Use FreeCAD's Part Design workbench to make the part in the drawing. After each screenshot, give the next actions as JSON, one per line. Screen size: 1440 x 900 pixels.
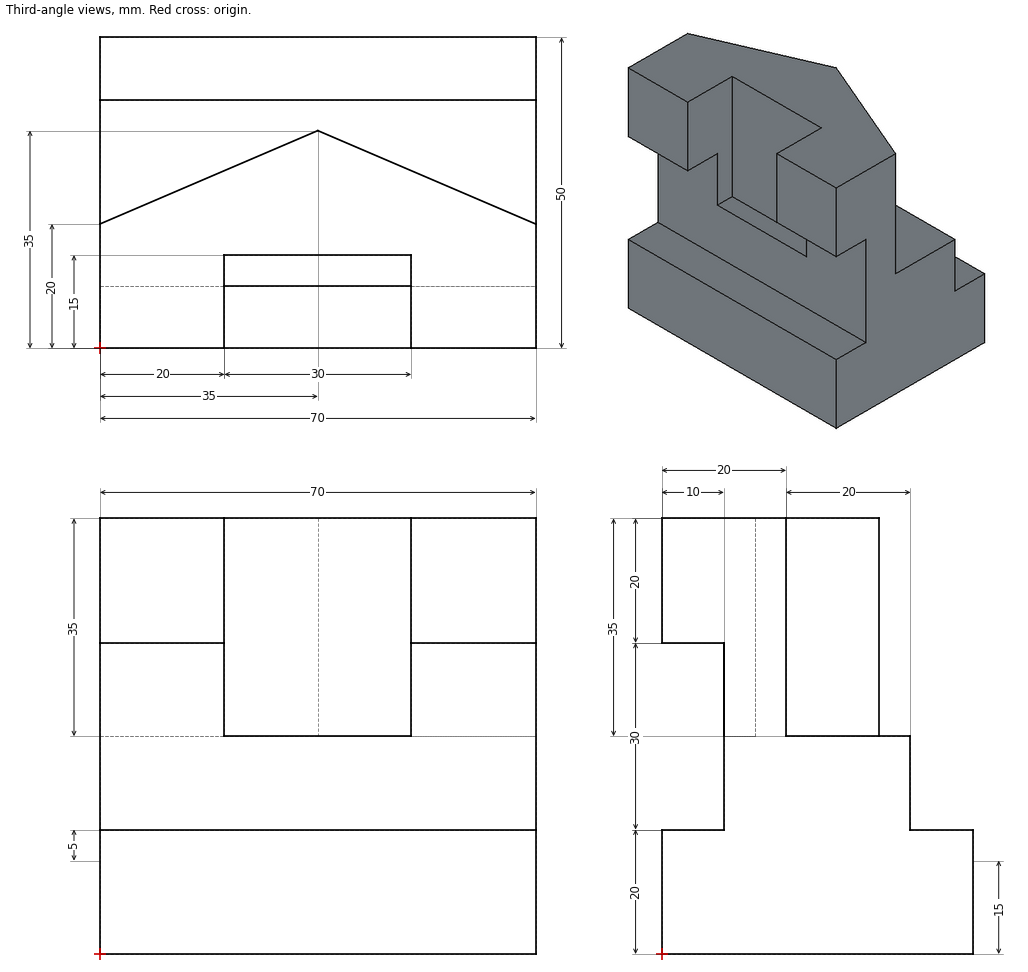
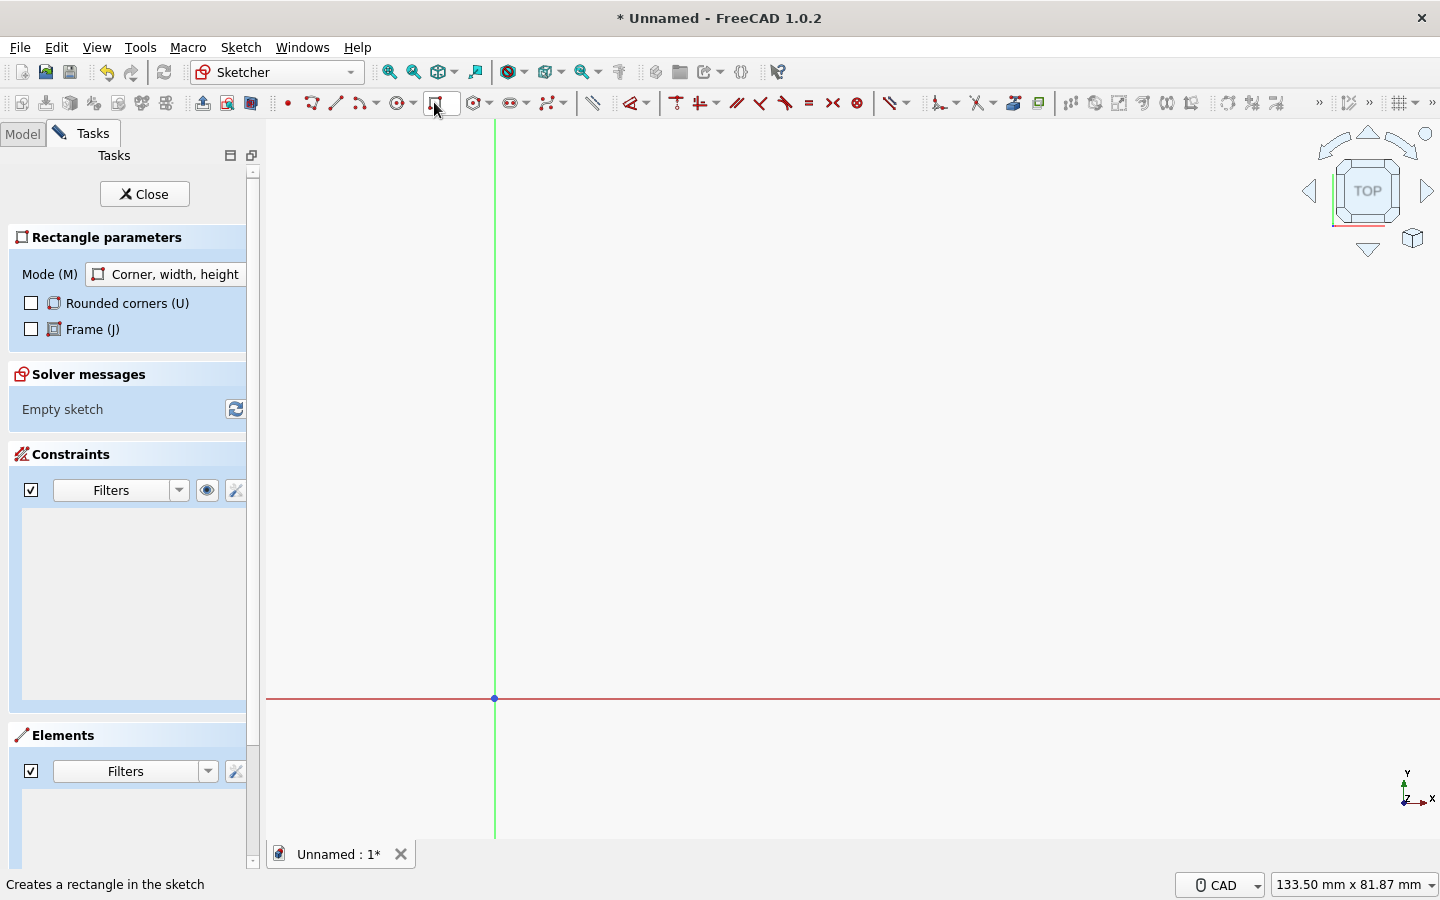
{"action": "left_click", "coordinate": [495, 699]}
{"action": "left_click", "coordinate": [1110, 259]}
{"action": "key", "text": "Escape"}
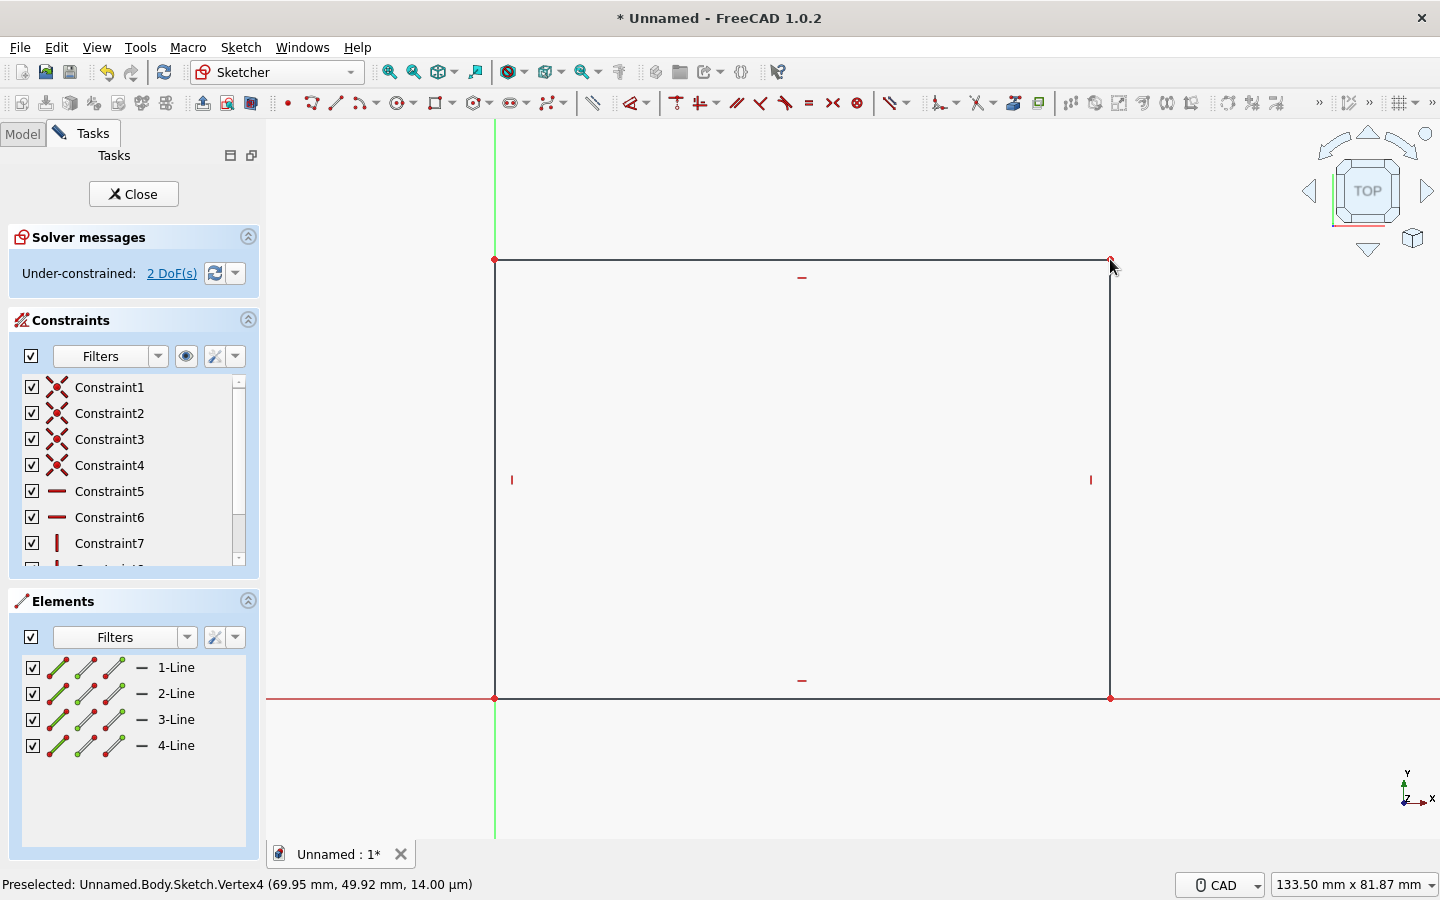
{"action": "left_click", "coordinate": [630, 104]}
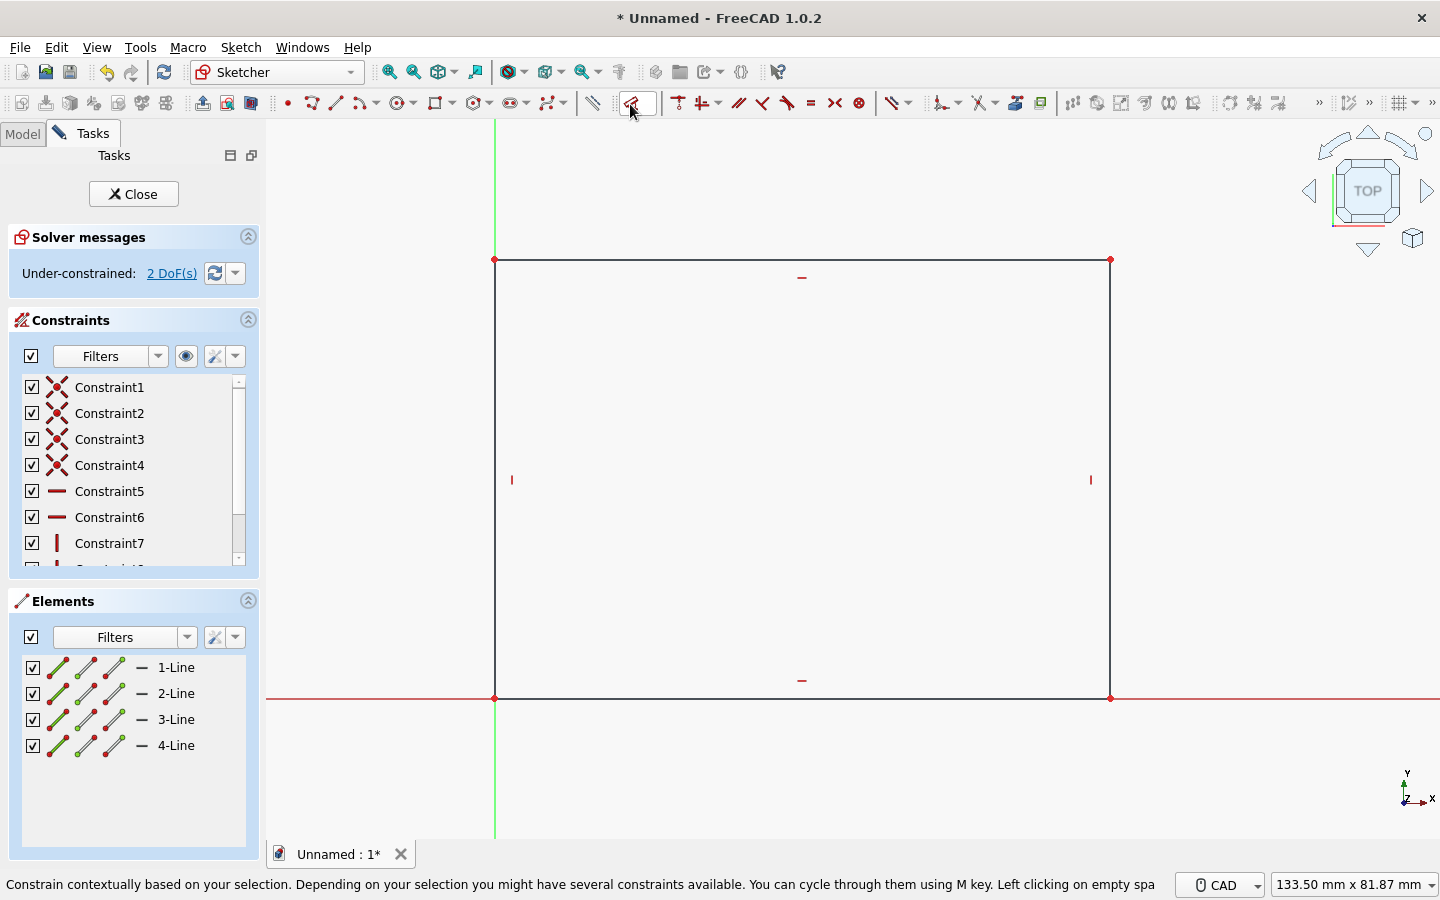
{"action": "left_click", "coordinate": [679, 699]}
{"action": "left_click", "coordinate": [802, 733]}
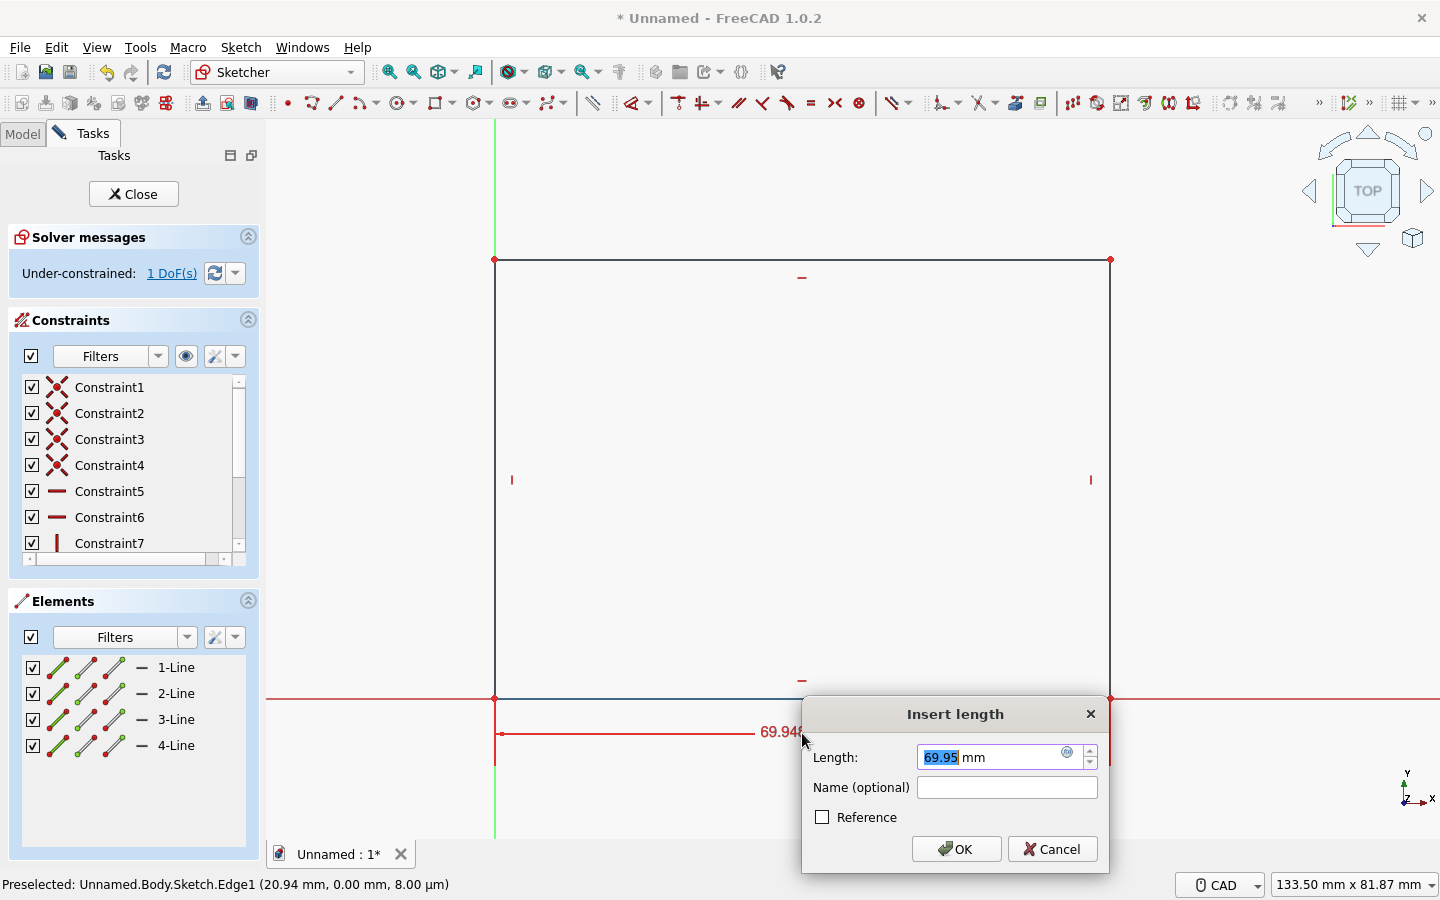
{"action": "type", "text": "70"}
{"action": "key", "text": "Return"}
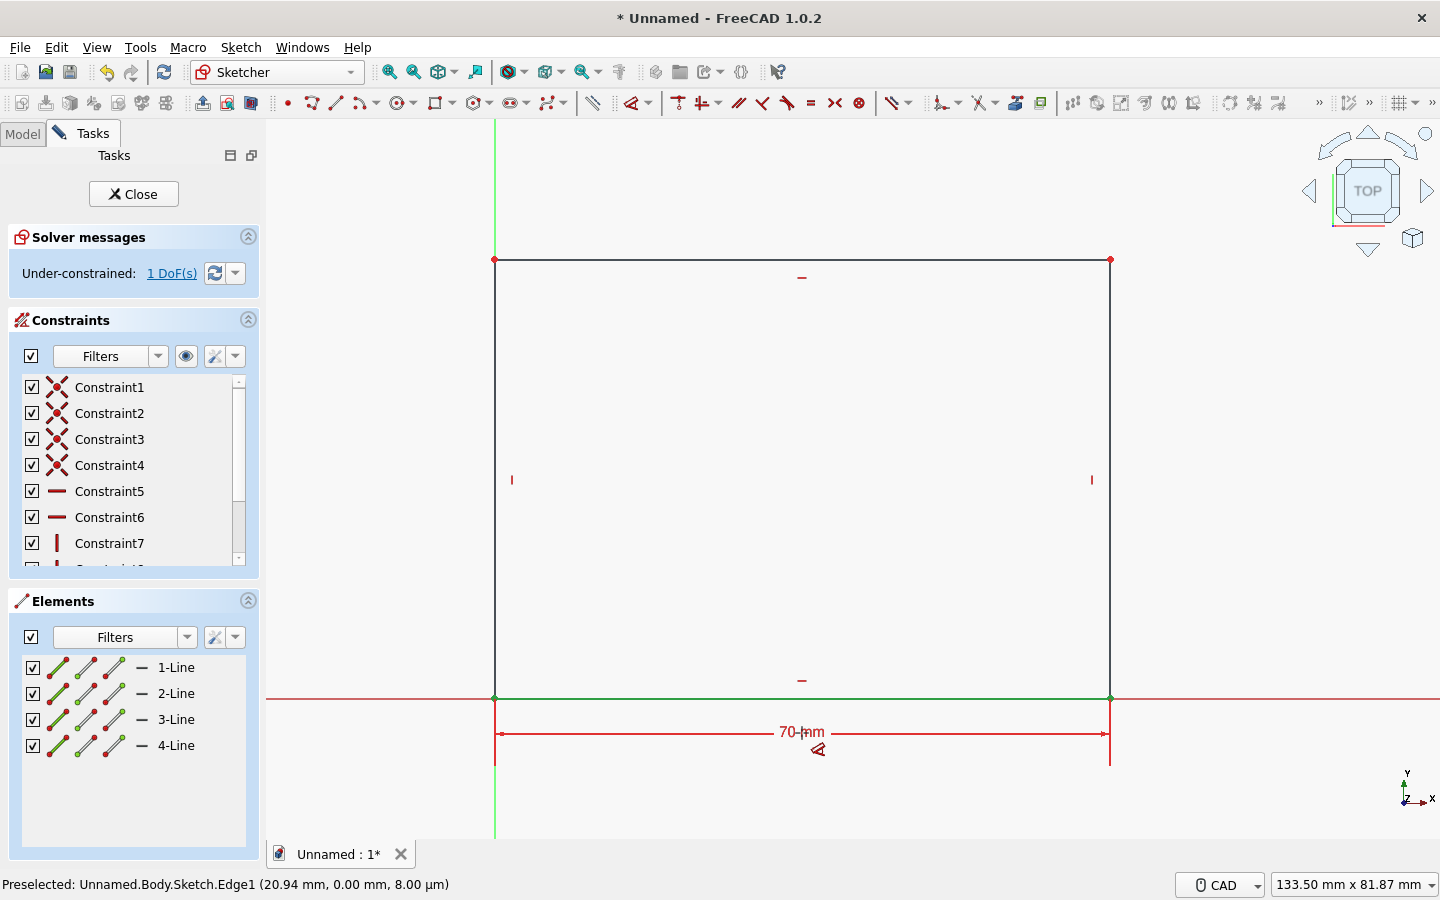
{"action": "left_click", "coordinate": [1110, 567]}
{"action": "left_click", "coordinate": [1144, 479]}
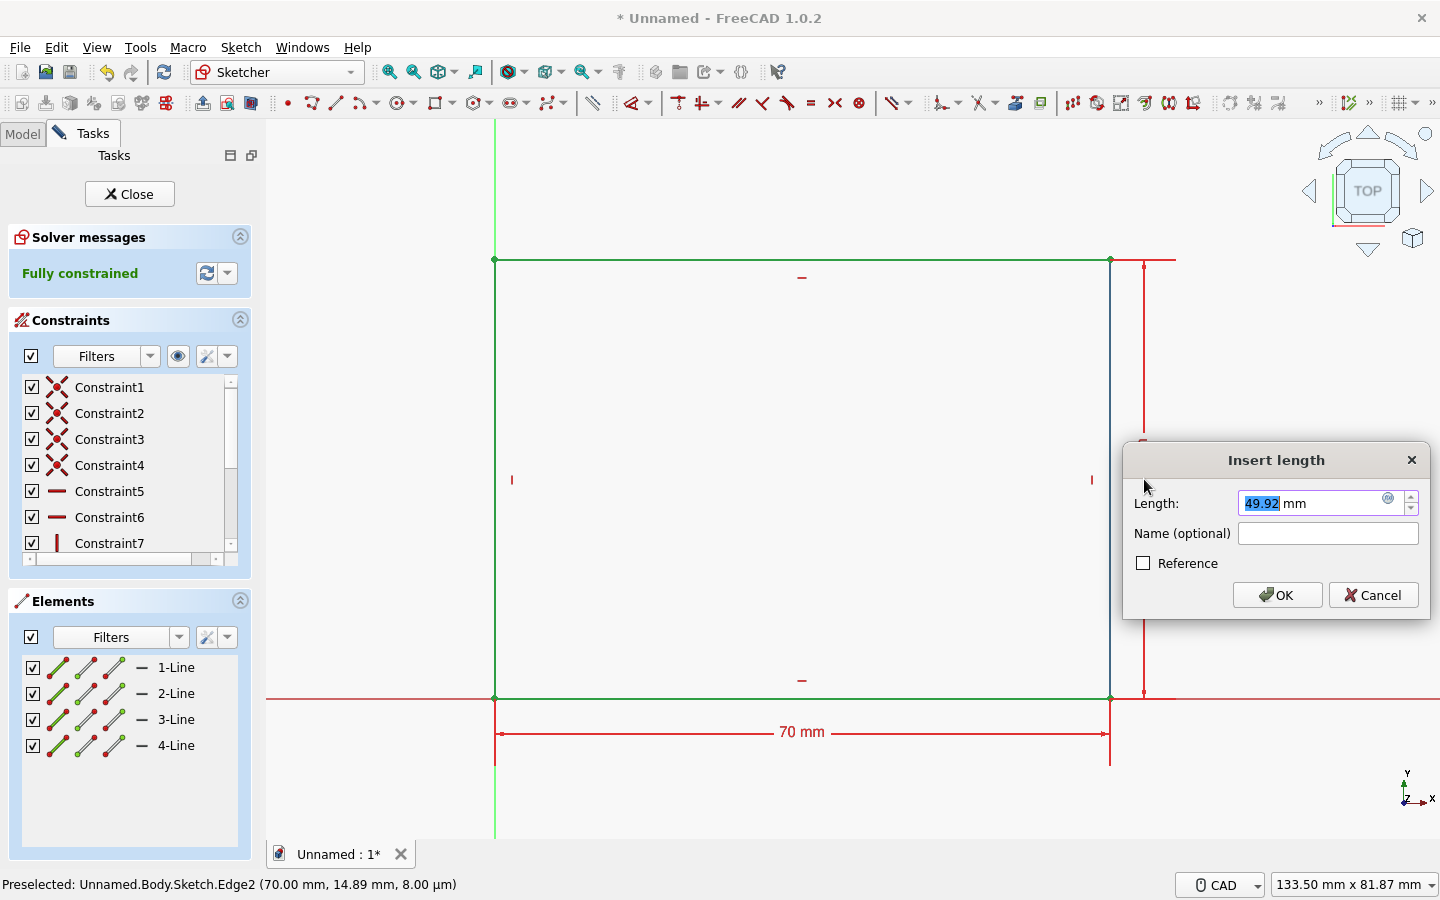
{"action": "type", "text": "50"}
{"action": "key", "text": "Return"}
{"action": "key", "text": "Escape"}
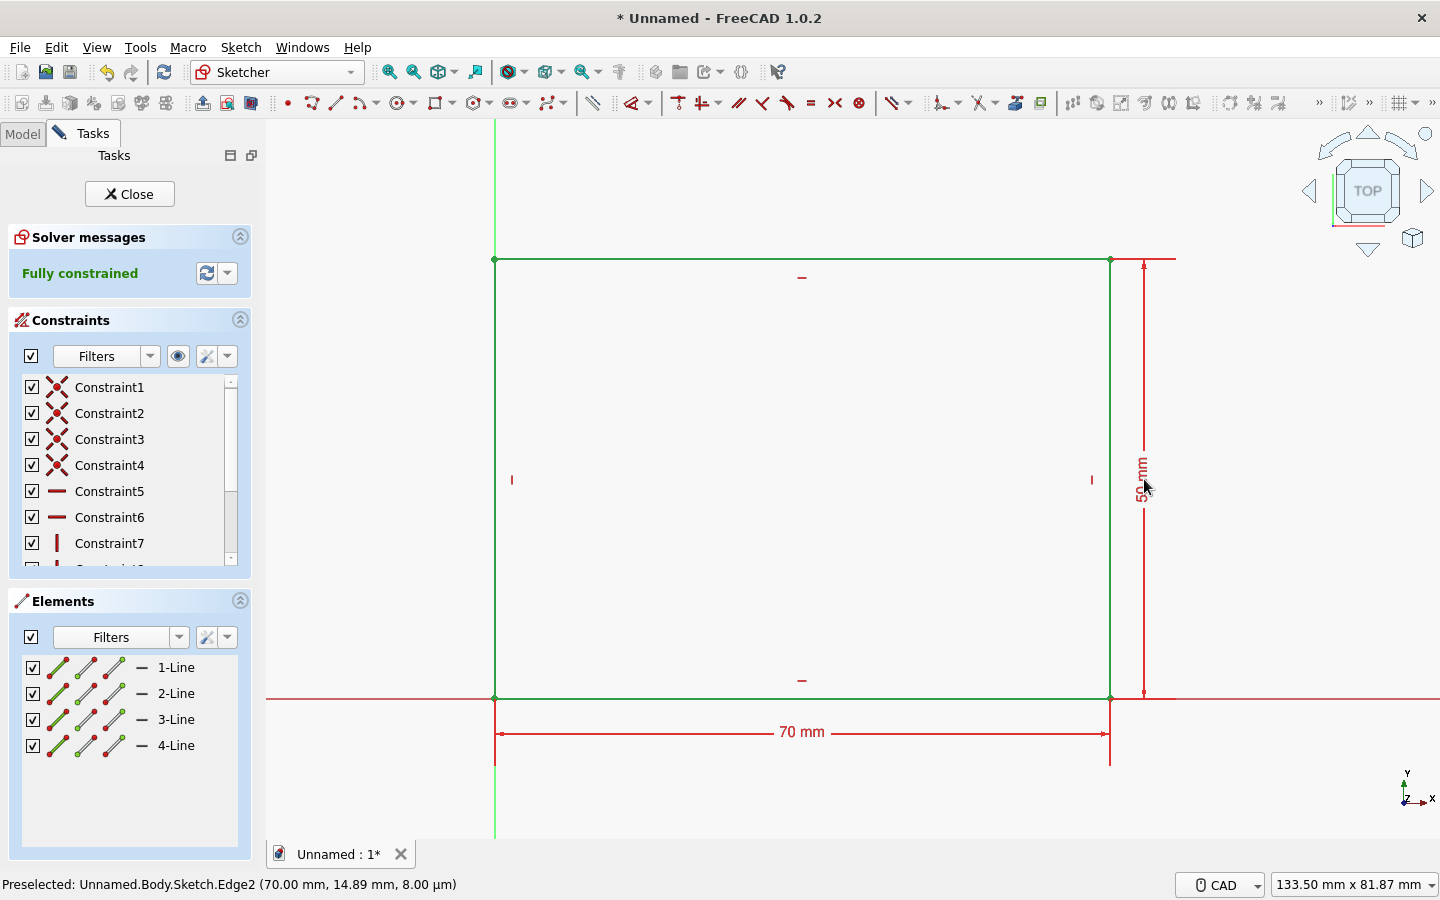
{"action": "left_click", "coordinate": [130, 194]}